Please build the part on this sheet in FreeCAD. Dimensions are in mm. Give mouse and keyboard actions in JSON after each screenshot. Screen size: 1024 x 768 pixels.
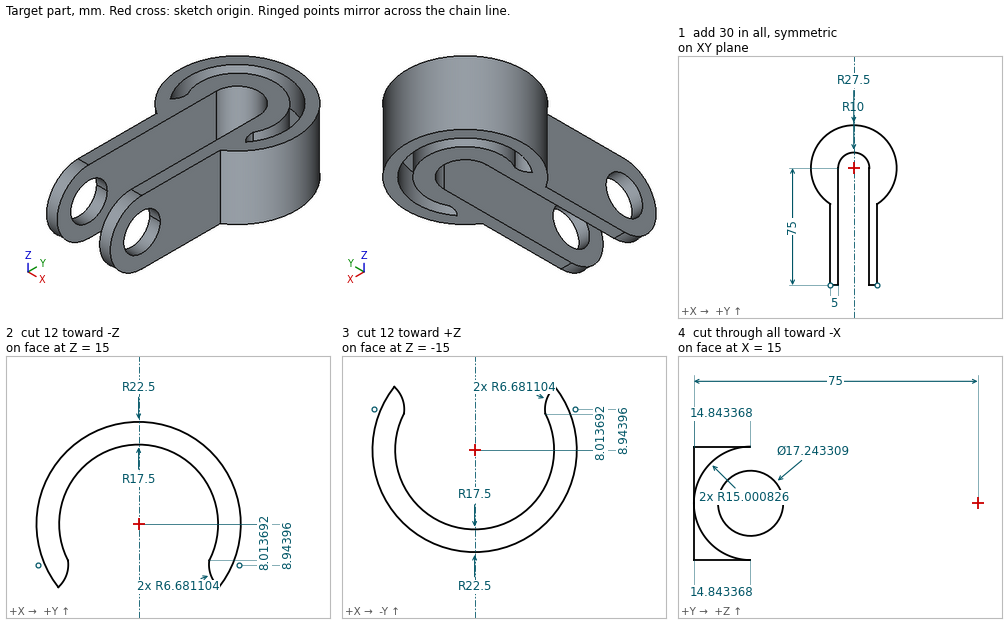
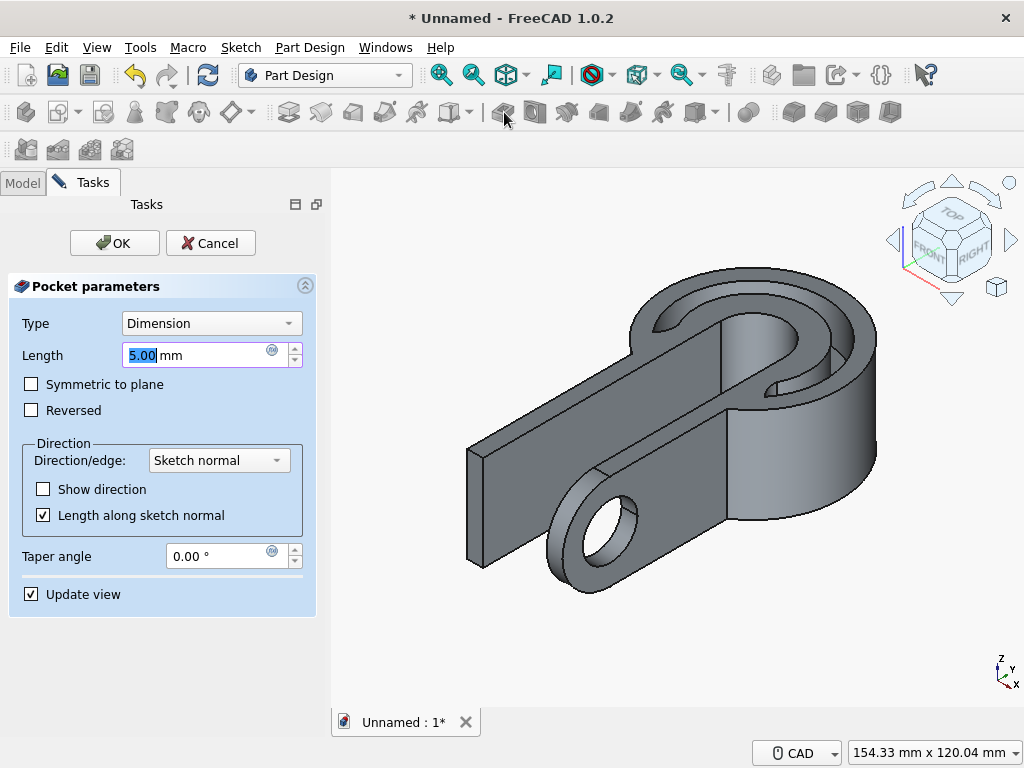
{"action": "left_click", "coordinate": [212, 324]}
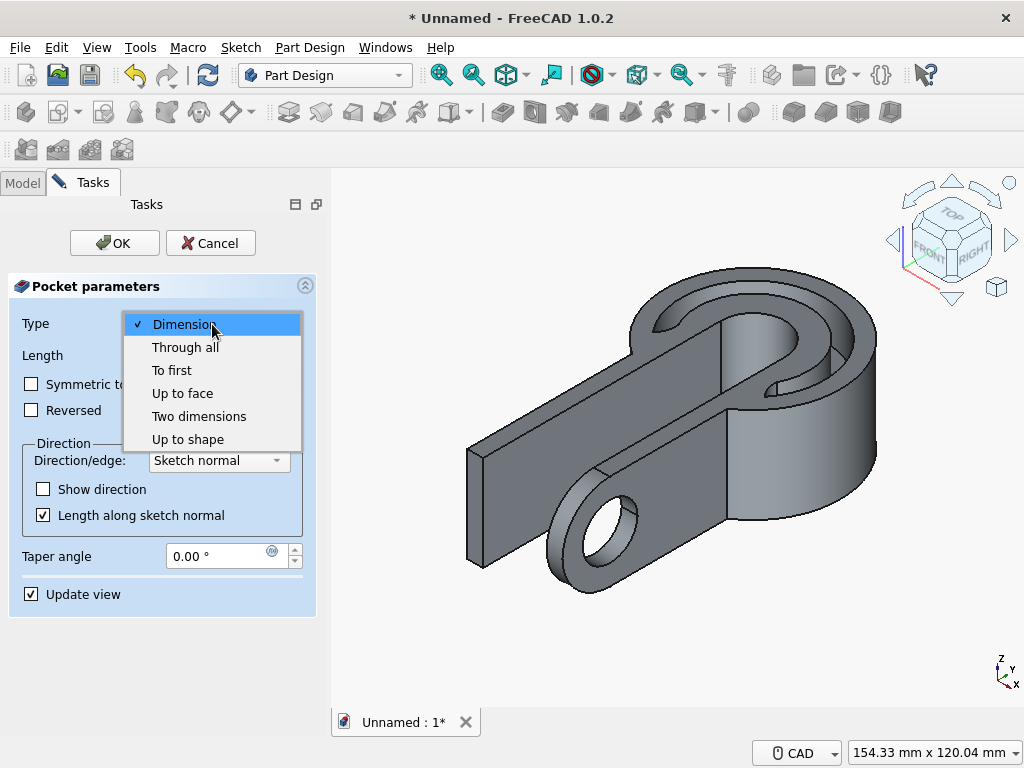
{"action": "left_click", "coordinate": [212, 348]}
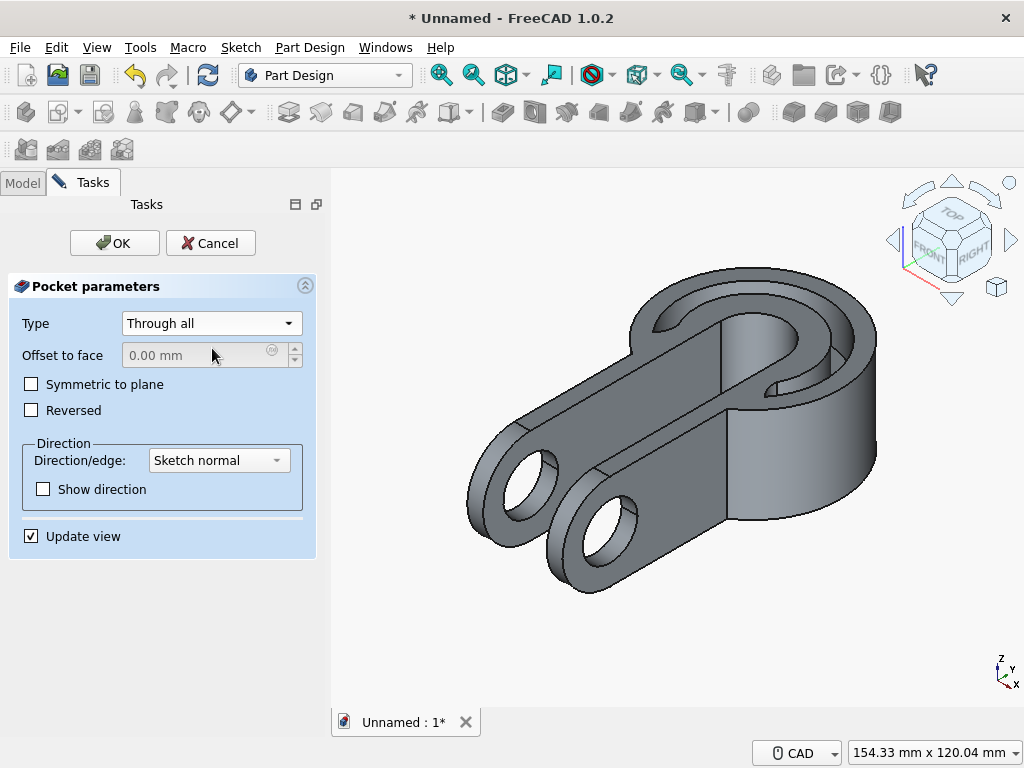
{"action": "left_click", "coordinate": [115, 243]}